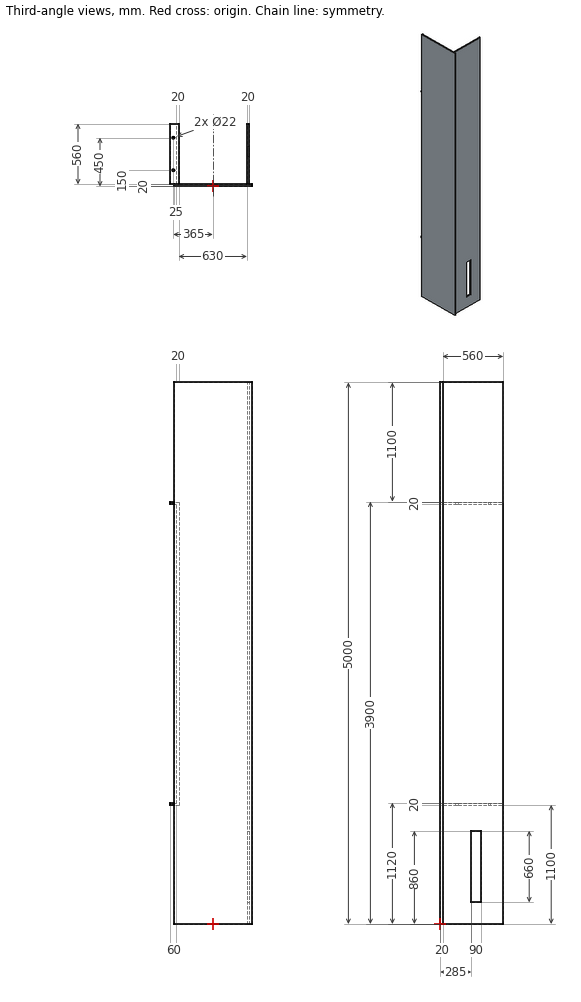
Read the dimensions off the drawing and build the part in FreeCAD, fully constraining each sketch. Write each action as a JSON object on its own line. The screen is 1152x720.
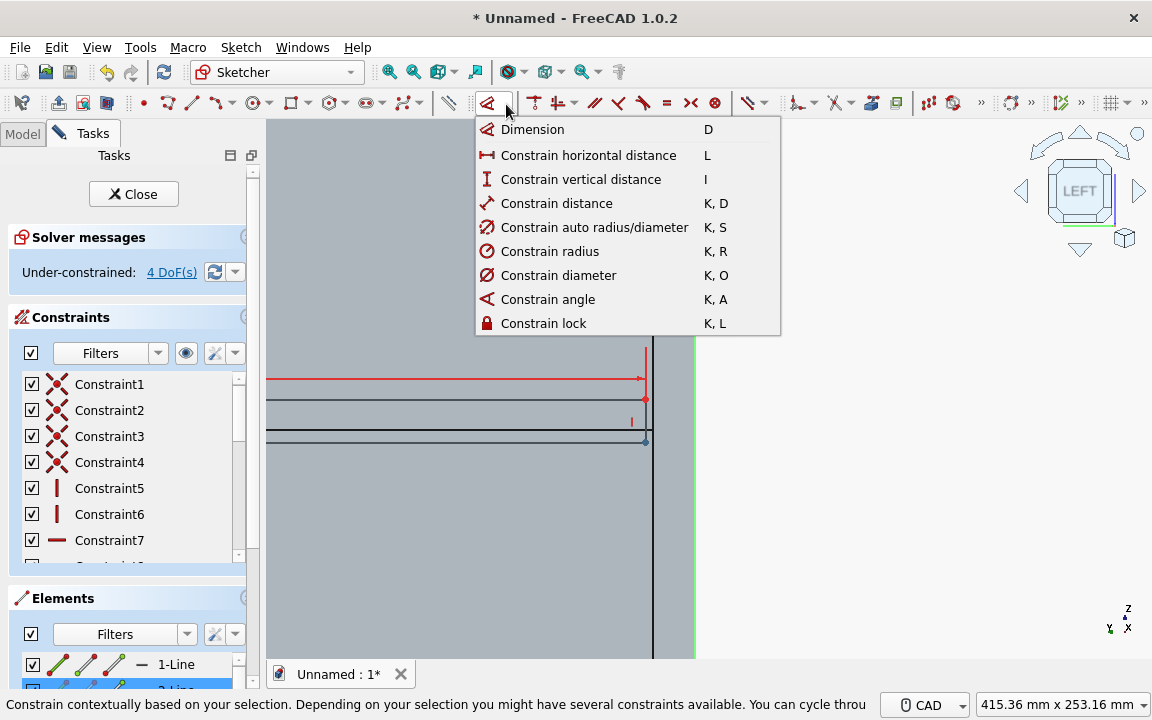
{"action": "left_click", "coordinate": [628, 155]}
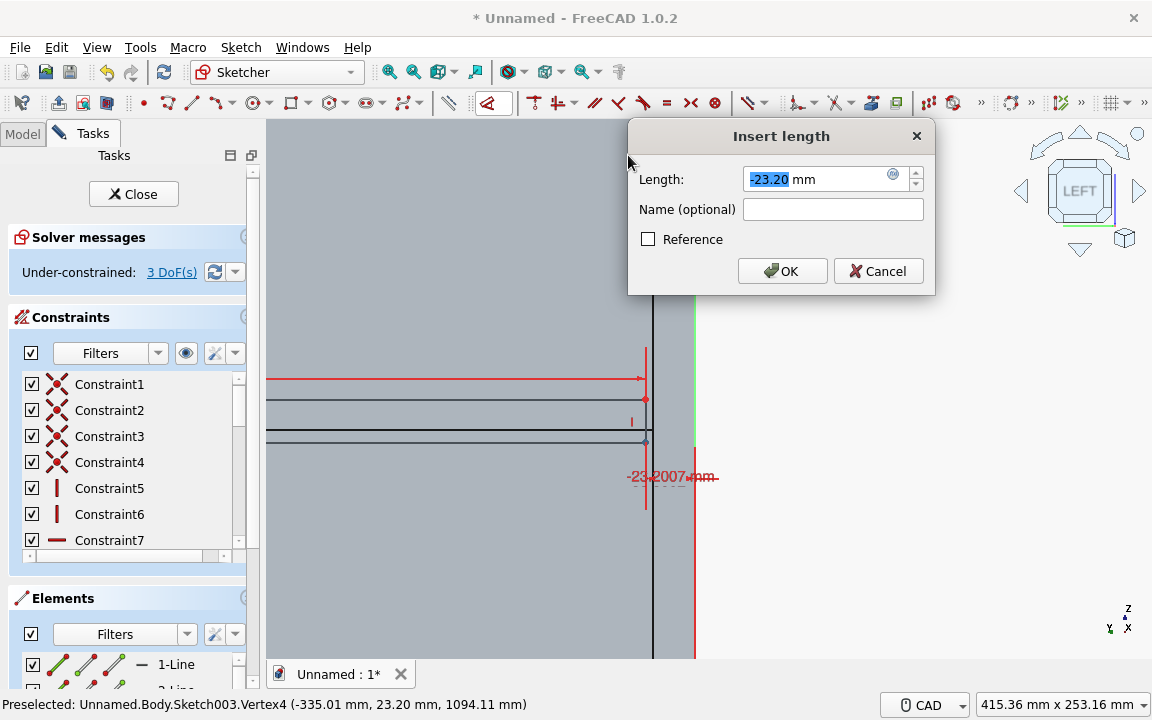
{"action": "type", "text": "-20"}
{"action": "key", "text": "Return"}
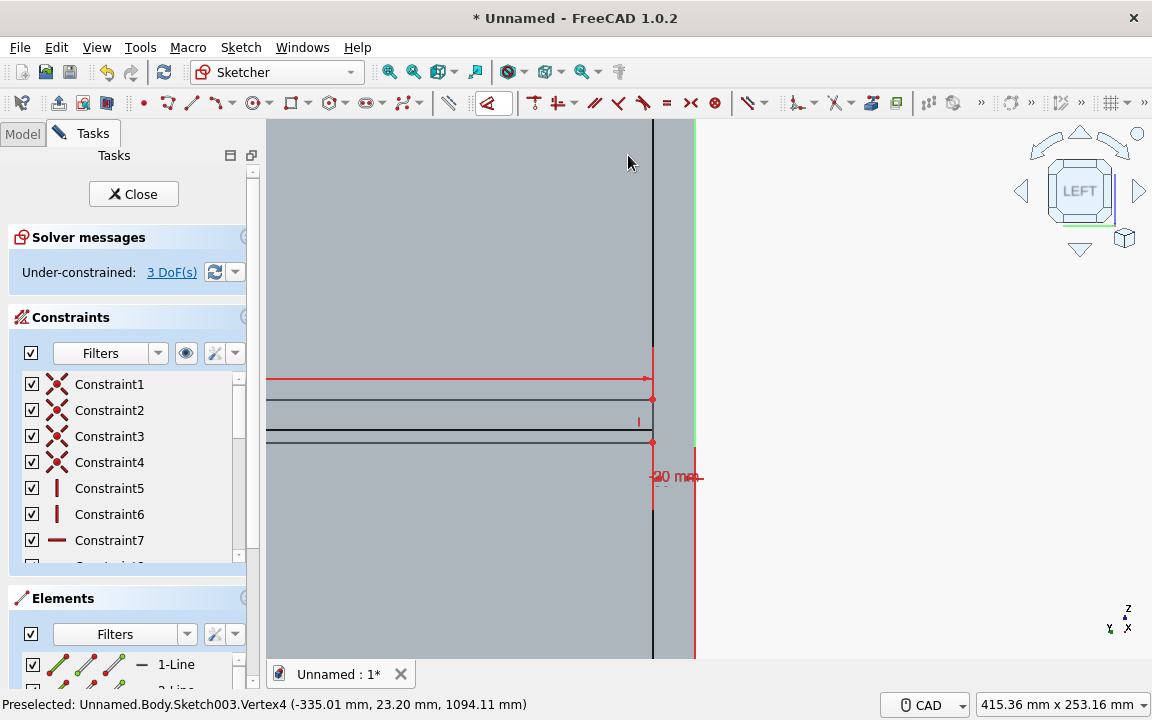
{"action": "scroll", "coordinate": [670, 482], "scroll_direction": "down", "scroll_amount": 15}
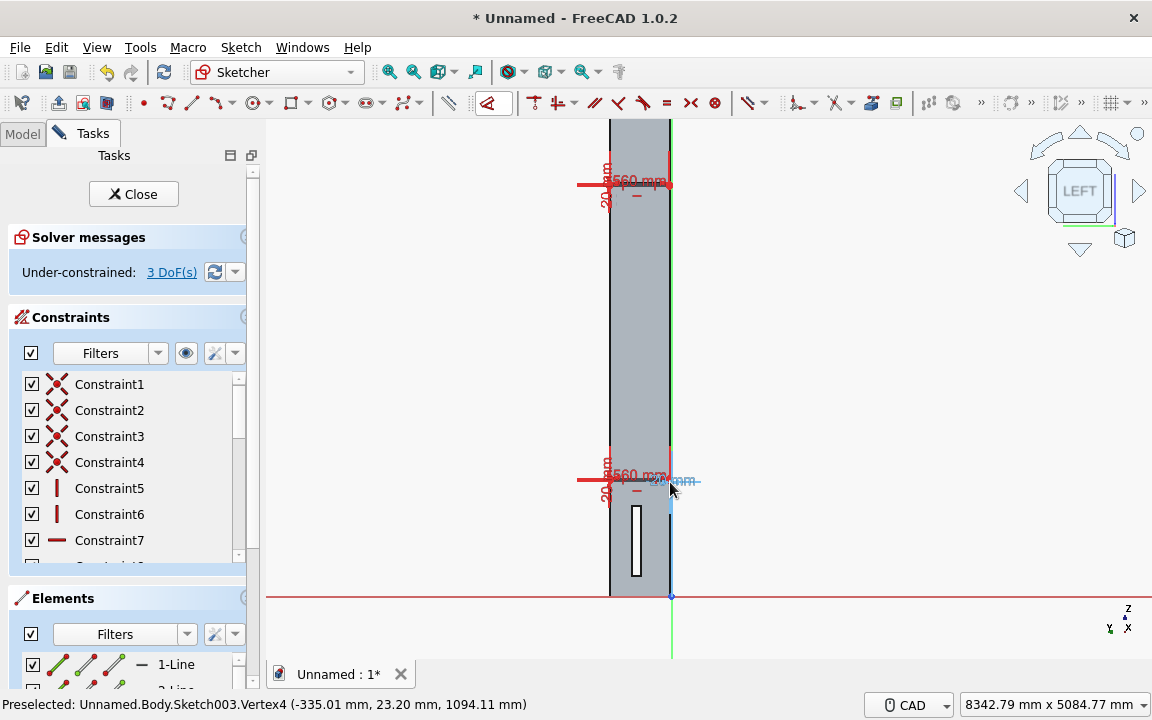
{"action": "scroll", "coordinate": [669, 186], "scroll_direction": "up", "scroll_amount": 15}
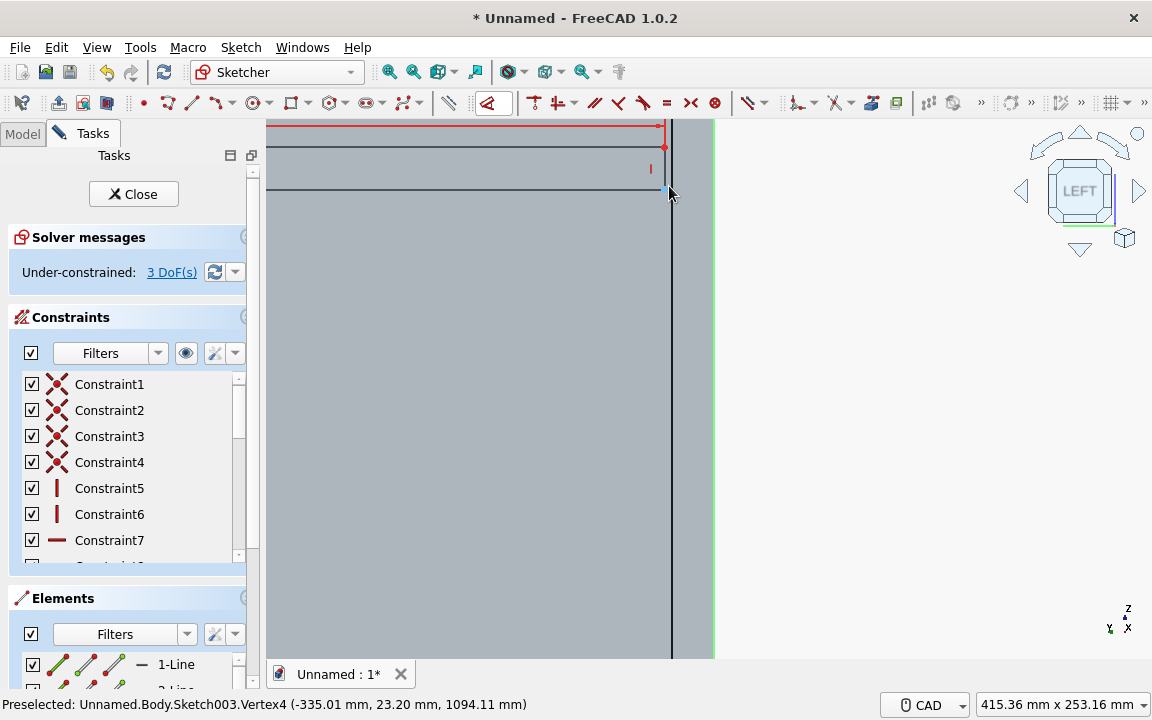
{"action": "left_click", "coordinate": [665, 190]}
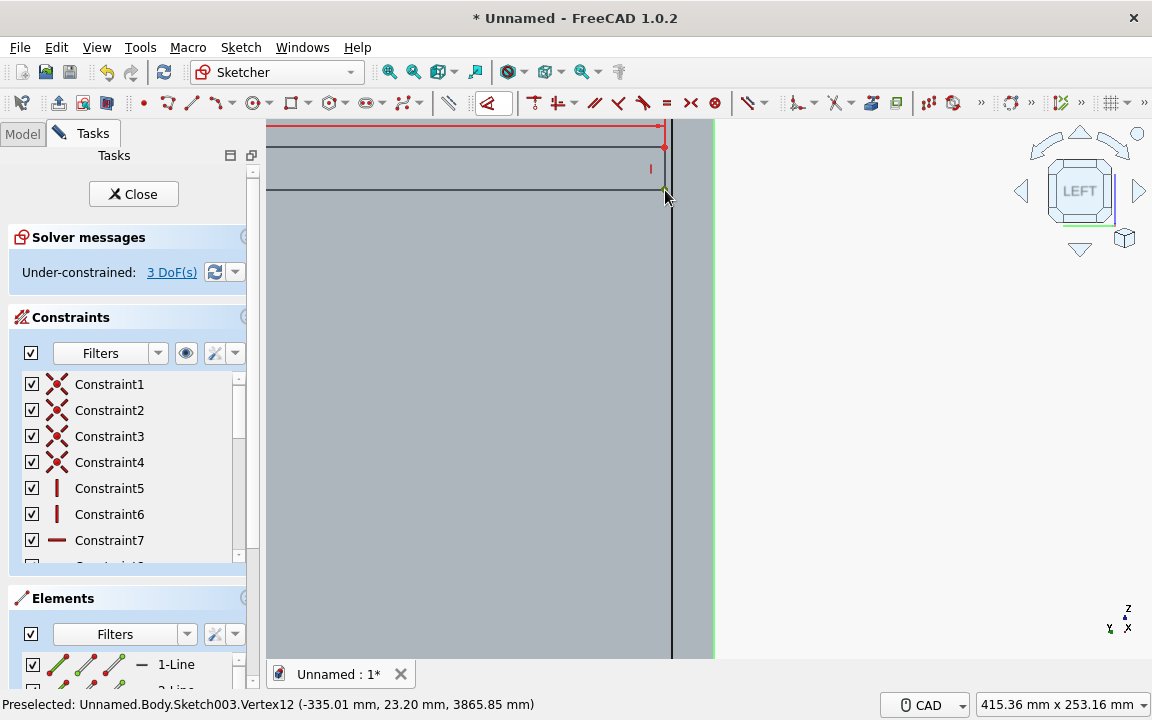
{"action": "key", "text": "l"}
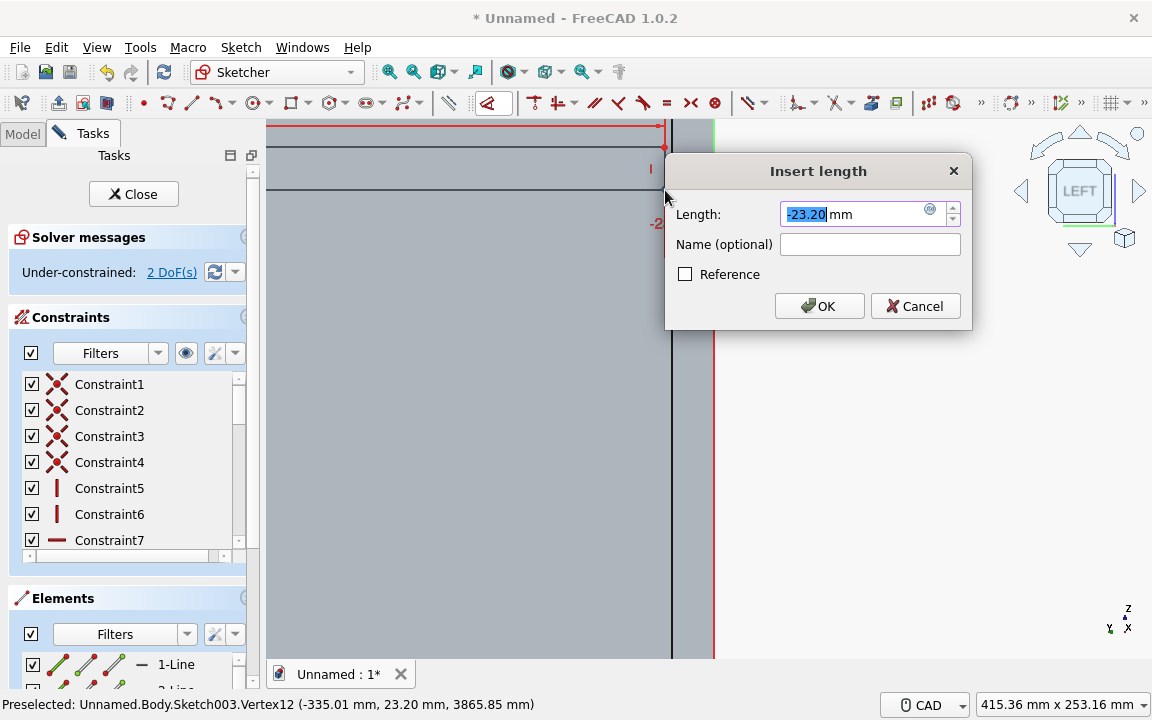
{"action": "type", "text": "-20"}
{"action": "key", "text": "Return"}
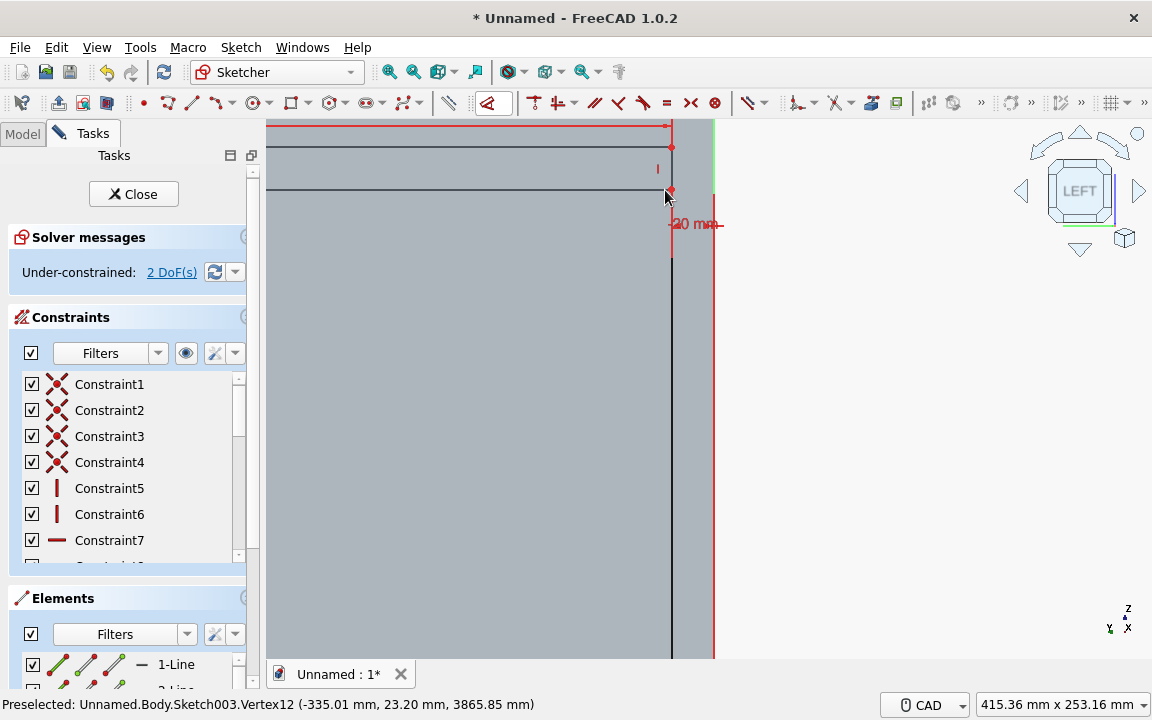
{"action": "scroll", "coordinate": [669, 185], "scroll_direction": "down", "scroll_amount": 15}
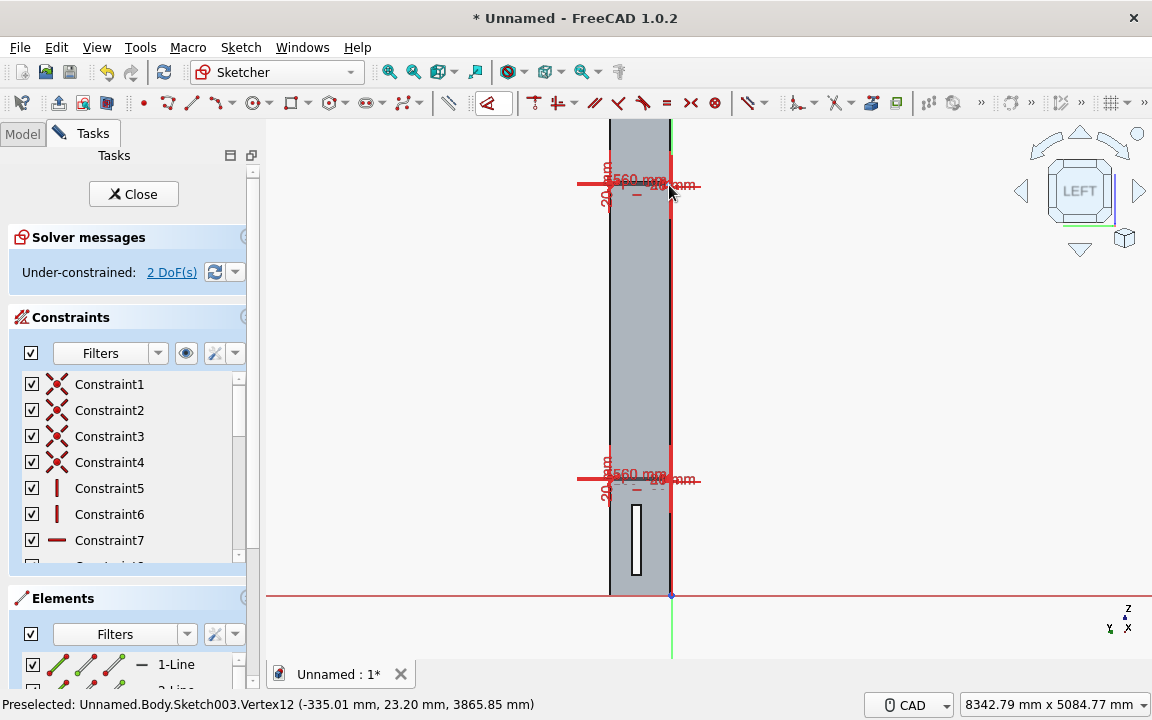
{"action": "scroll", "coordinate": [610, 478], "scroll_direction": "up", "scroll_amount": 9}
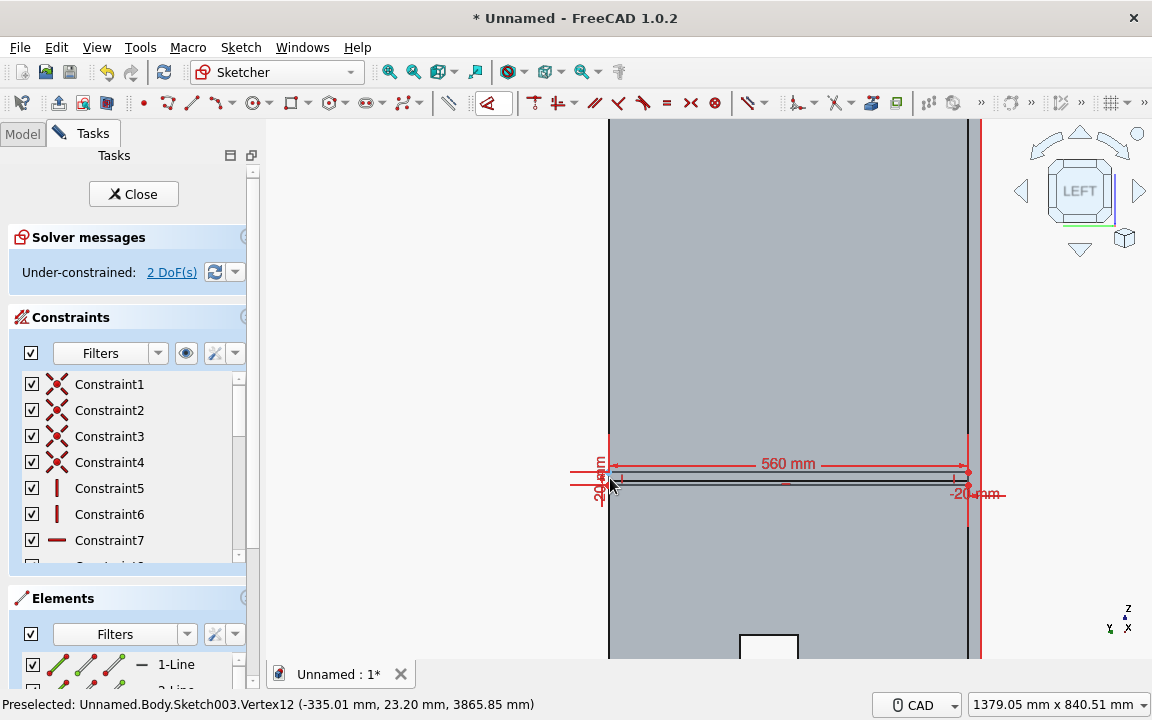
{"action": "left_click", "coordinate": [609, 472]}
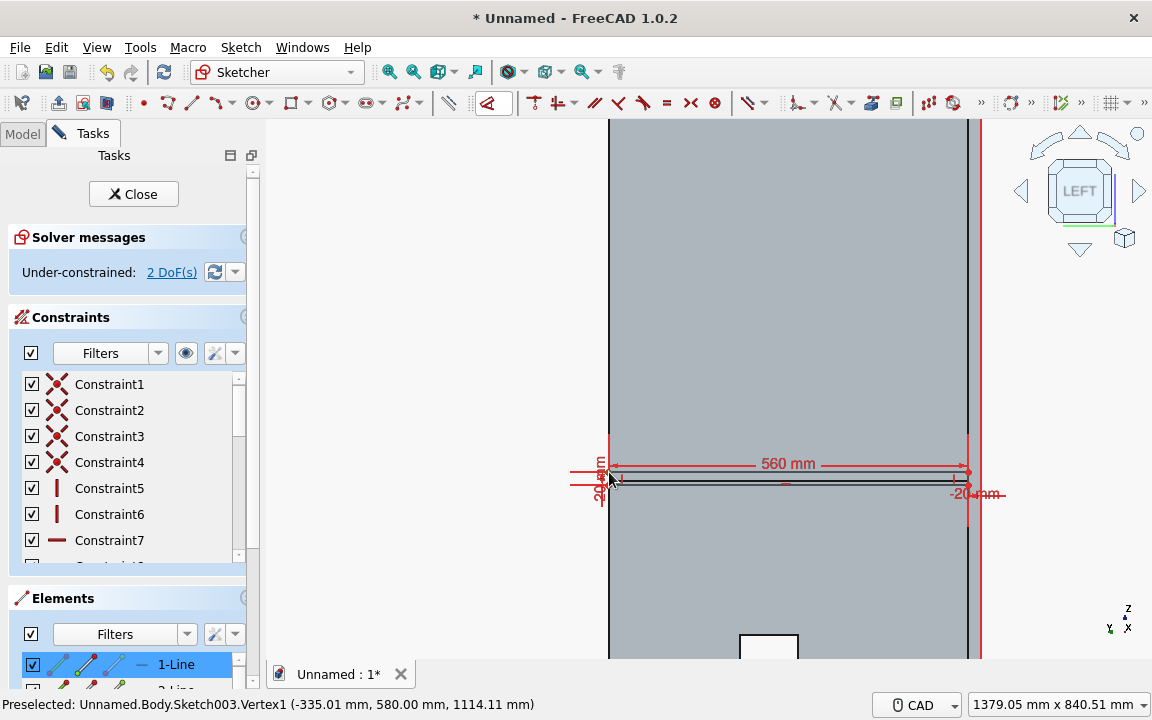
{"action": "key", "text": "i"}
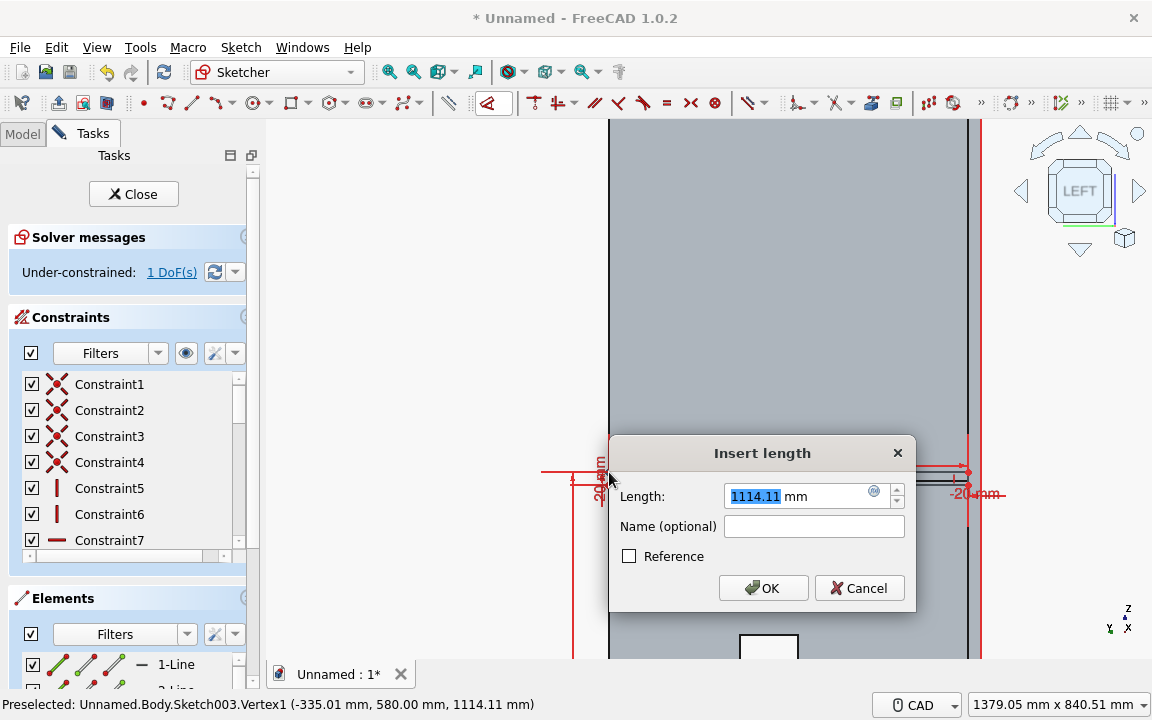
{"action": "type", "text": "1120"}
{"action": "key", "text": "Return"}